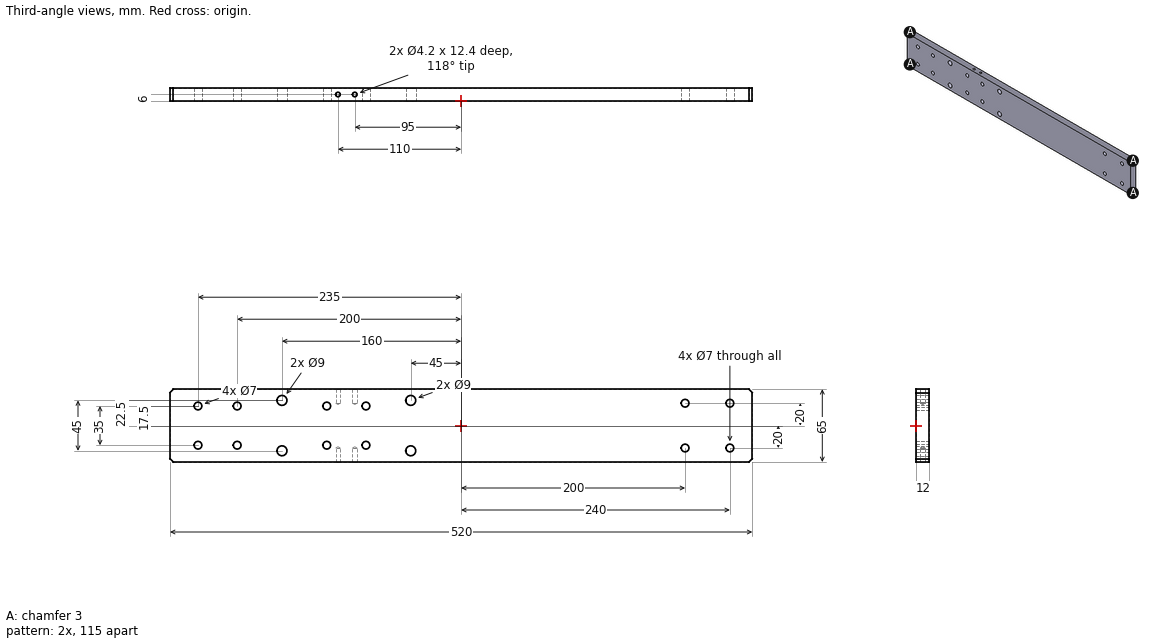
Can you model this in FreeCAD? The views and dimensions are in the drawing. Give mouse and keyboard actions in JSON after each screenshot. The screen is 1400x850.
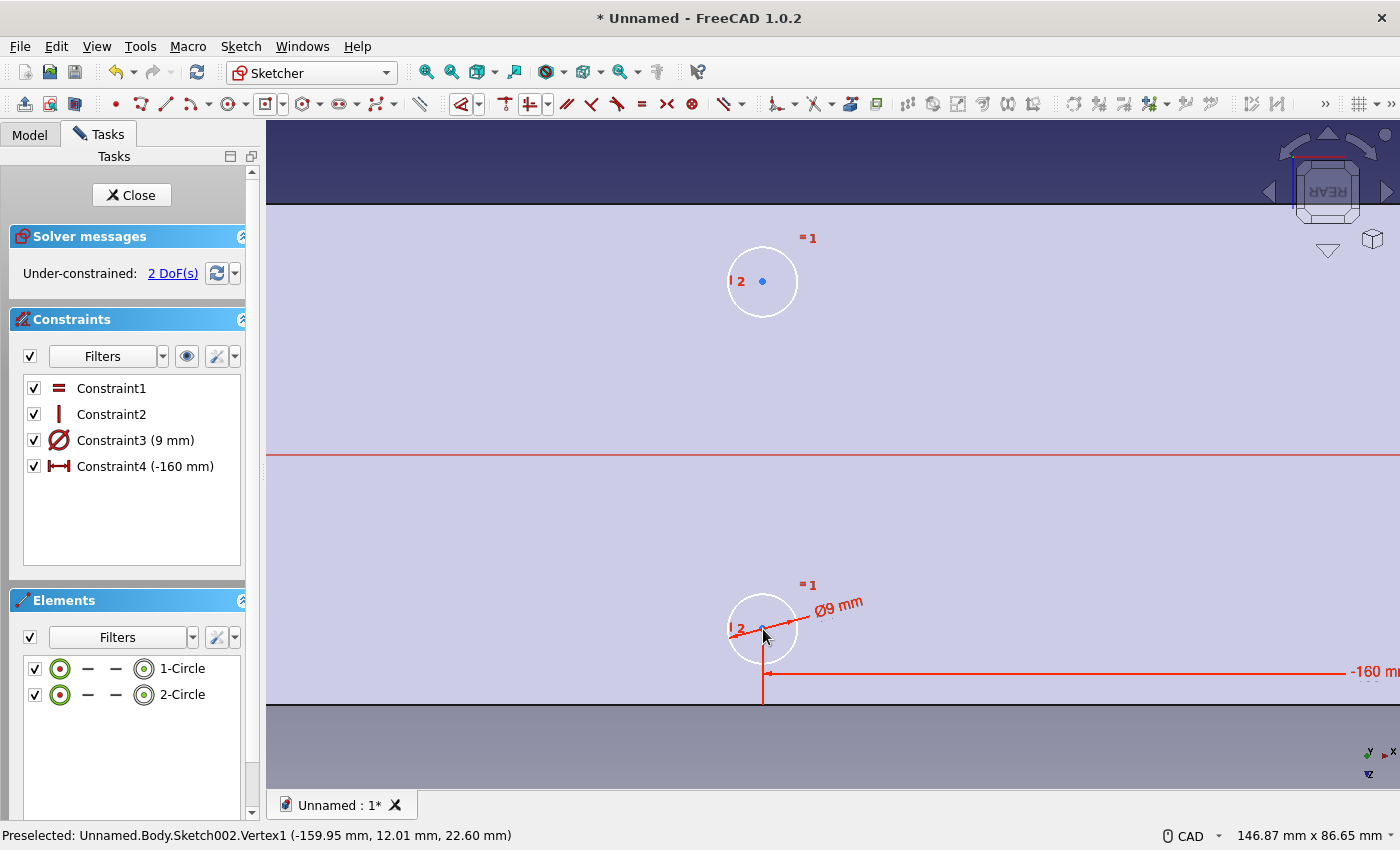
{"action": "left_click", "coordinate": [763, 629]}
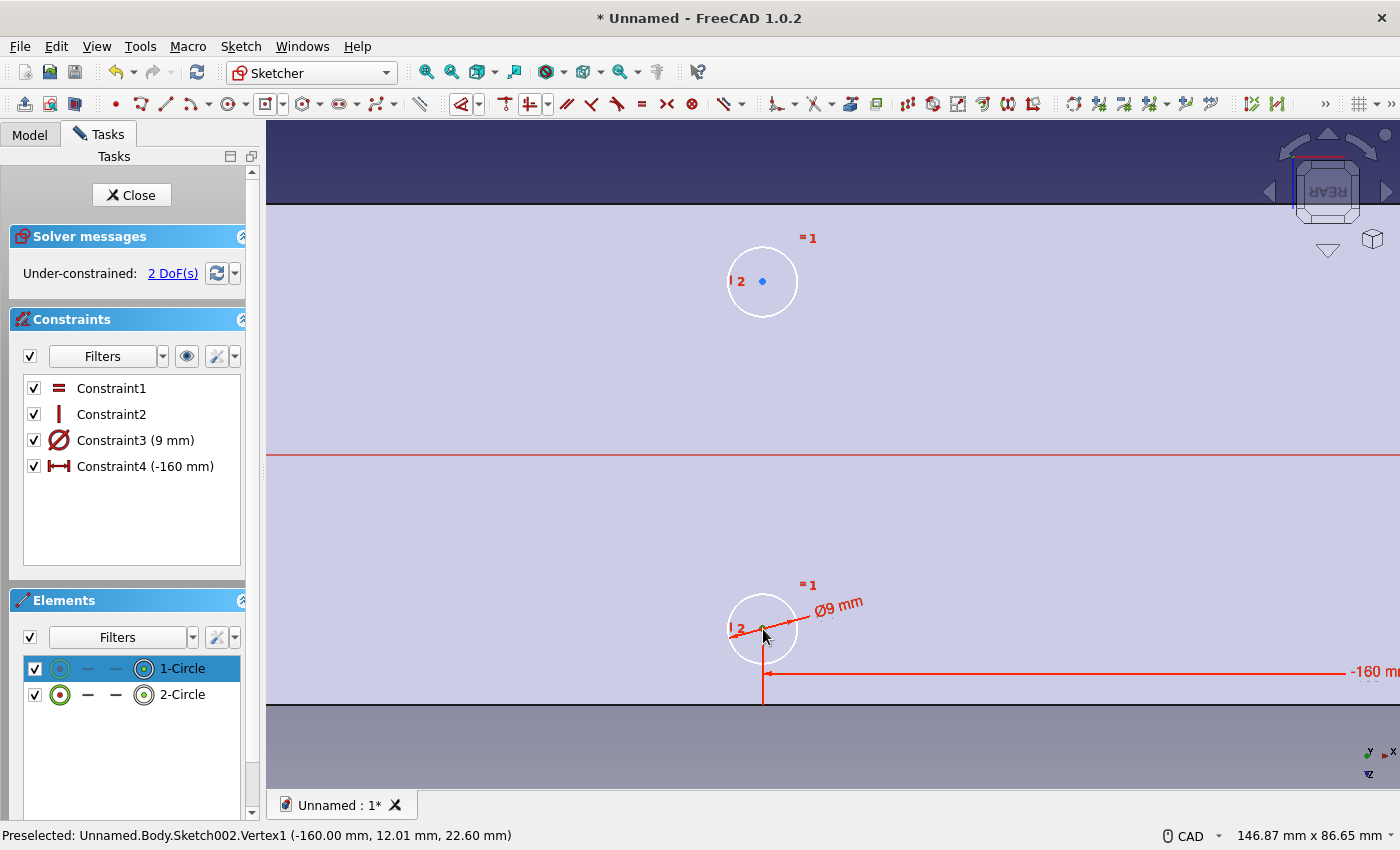
{"action": "left_click", "coordinate": [763, 282]}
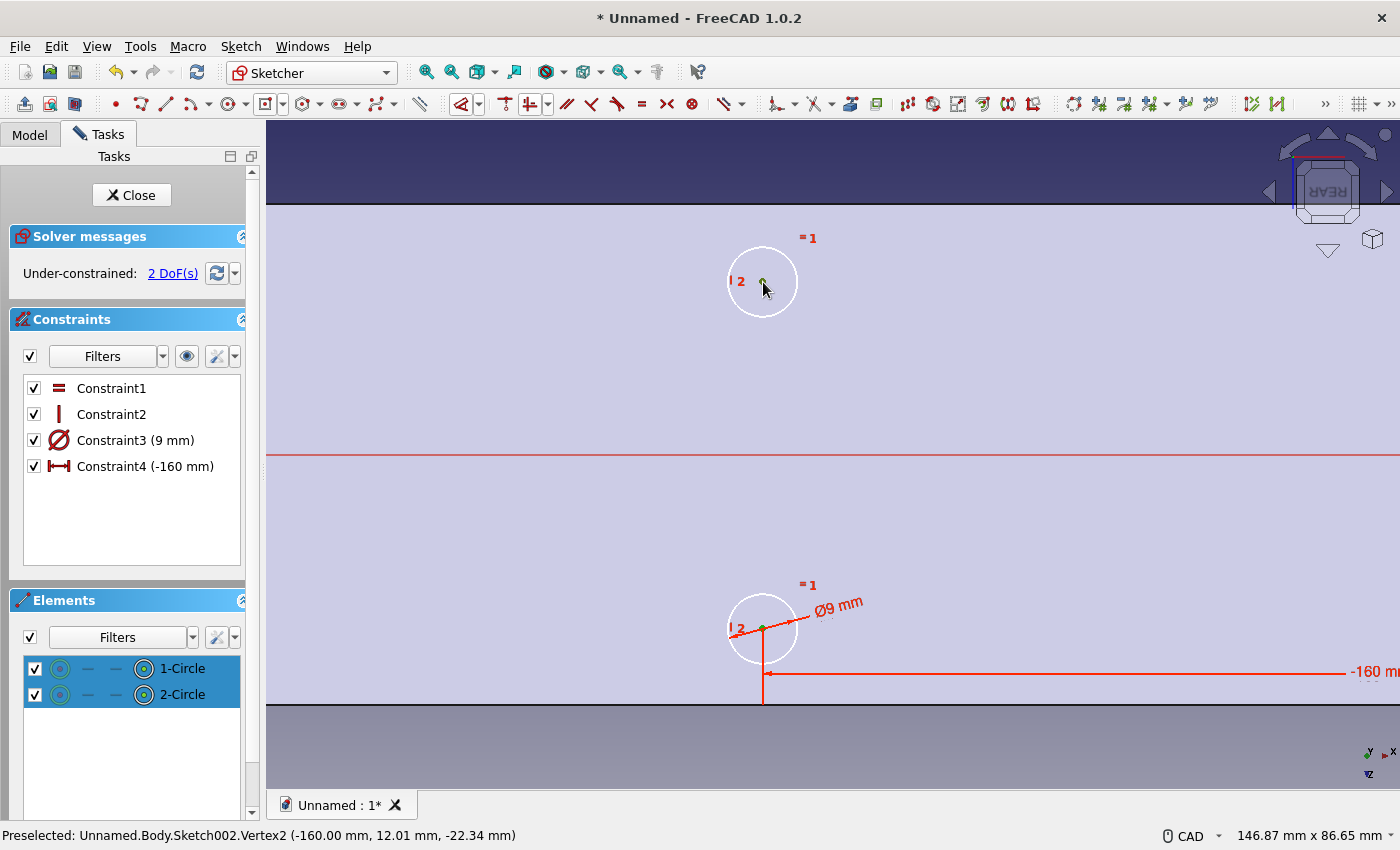
{"action": "left_click", "coordinate": [478, 104]}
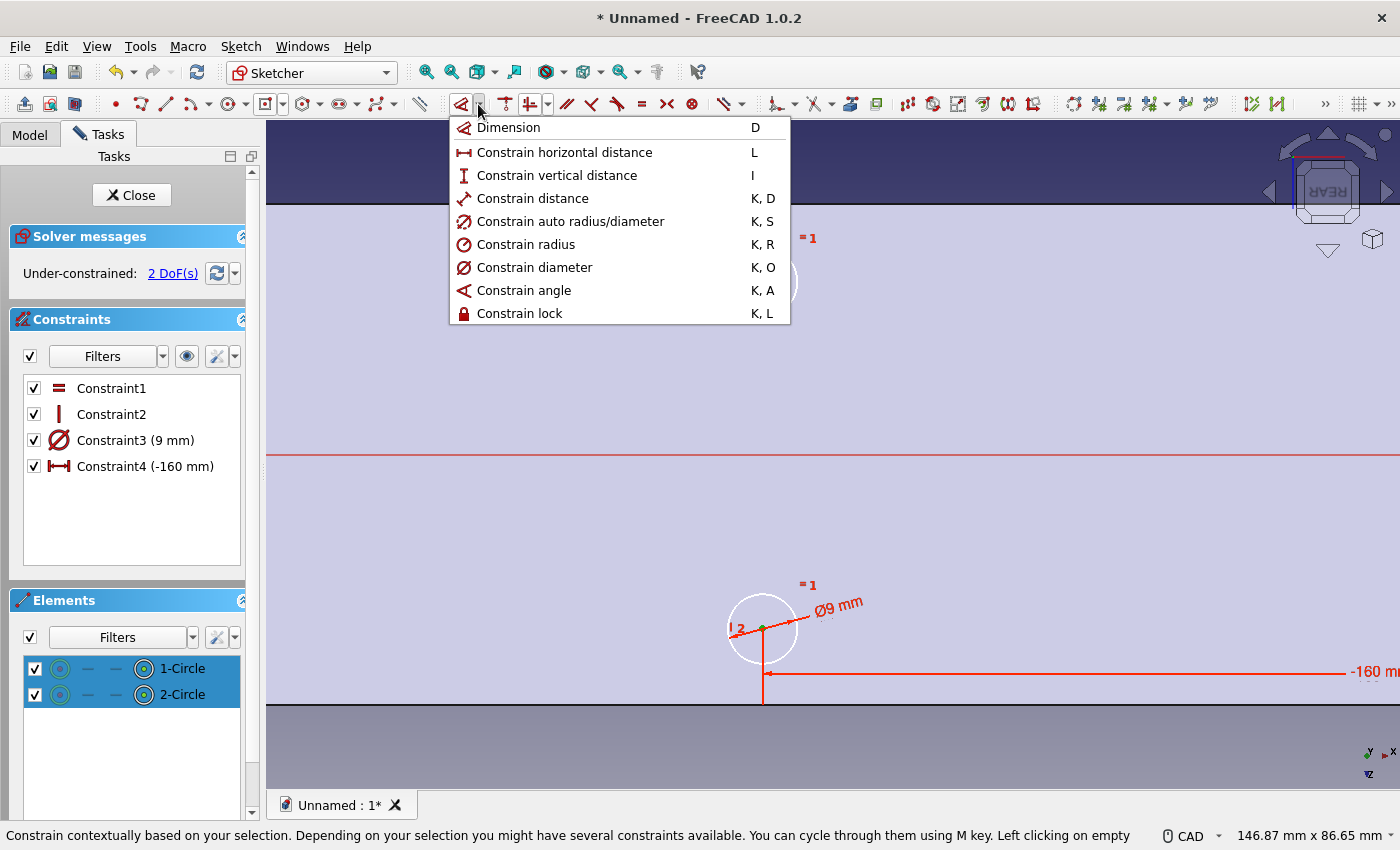
{"action": "left_click", "coordinate": [620, 176]}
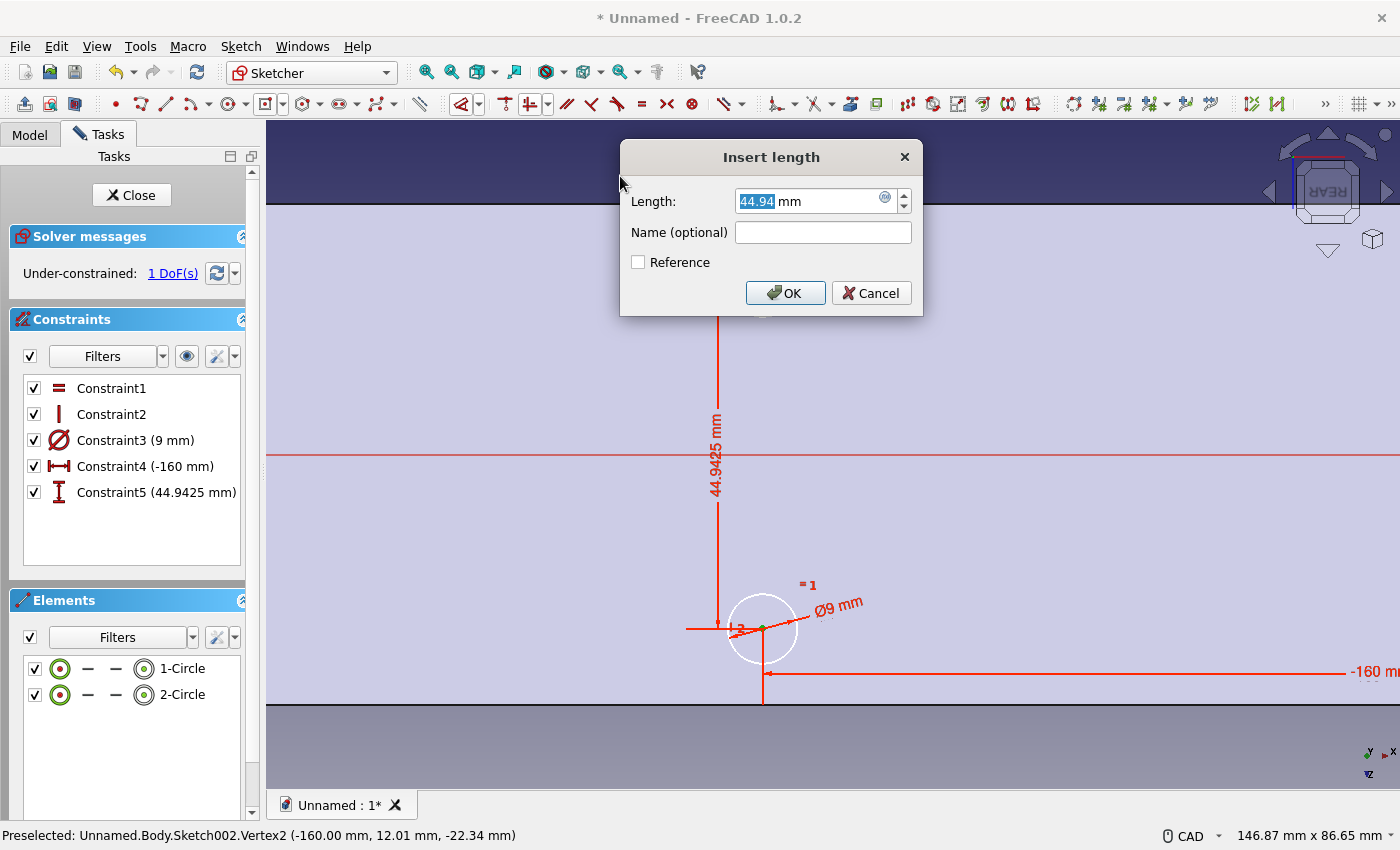
{"action": "type", "text": "45"}
{"action": "key", "text": "Return"}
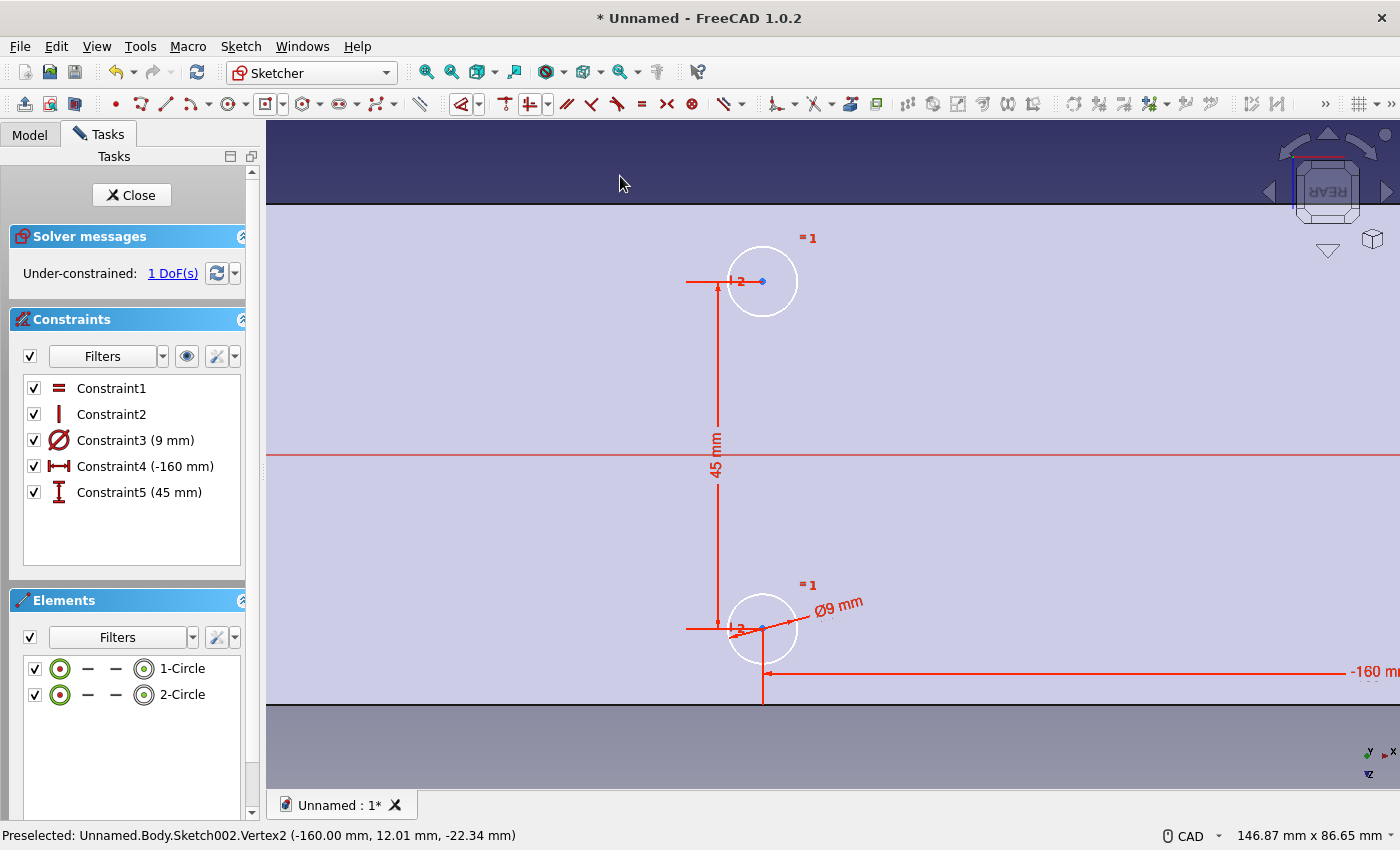
{"action": "left_click", "coordinate": [763, 629]}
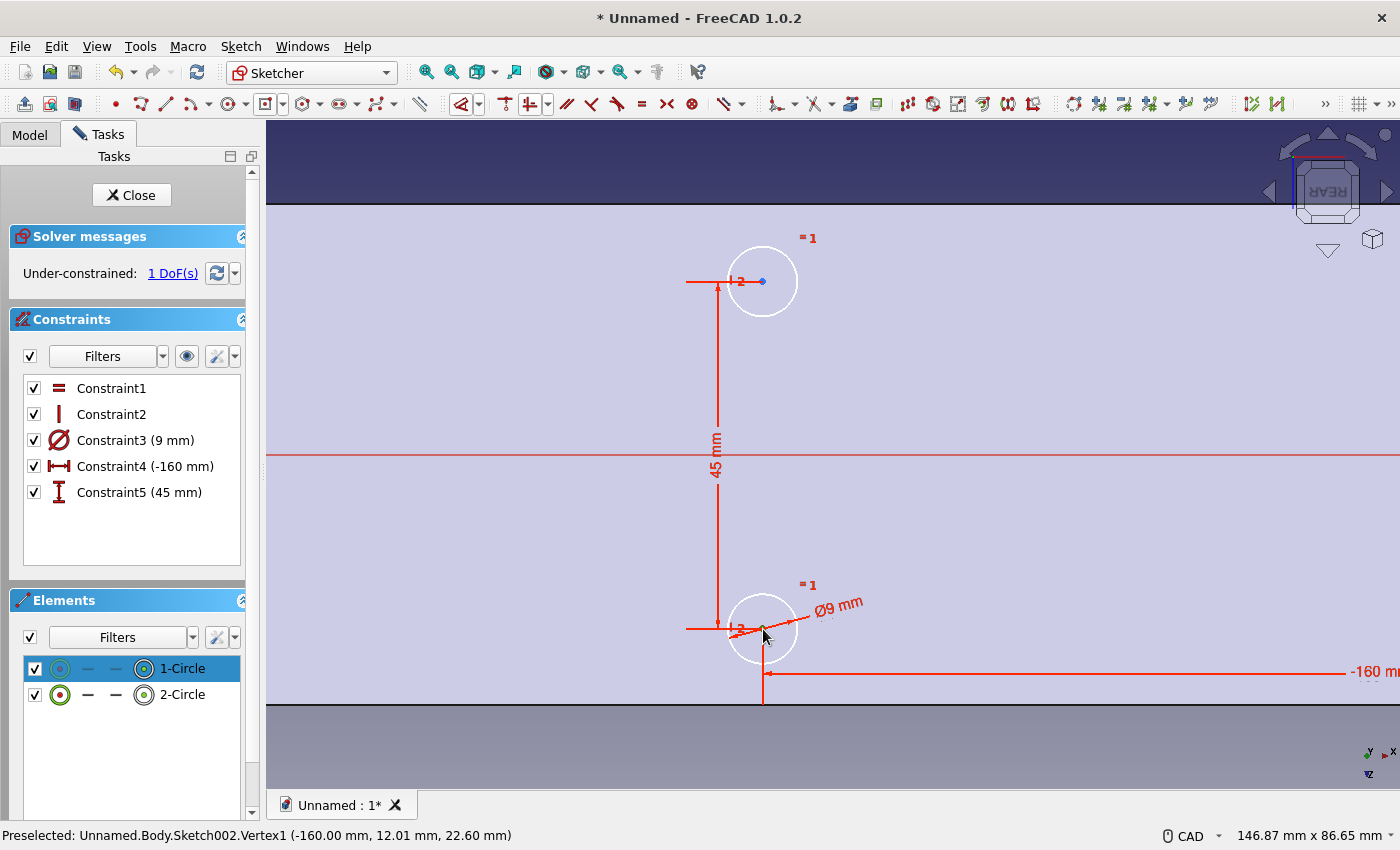
{"action": "key", "text": "i"}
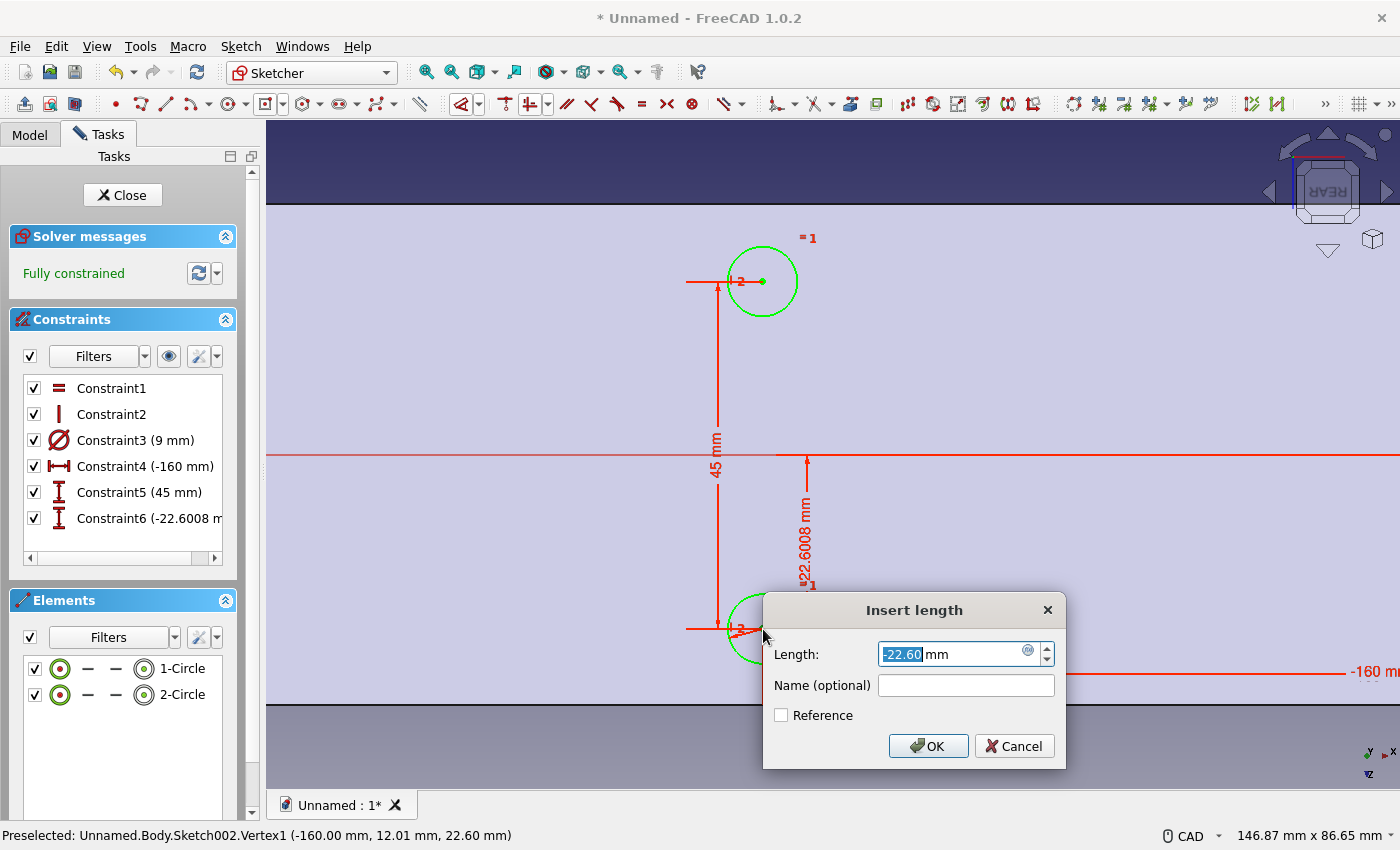
{"action": "type", "text": "-22.5"}
{"action": "key", "text": "Return"}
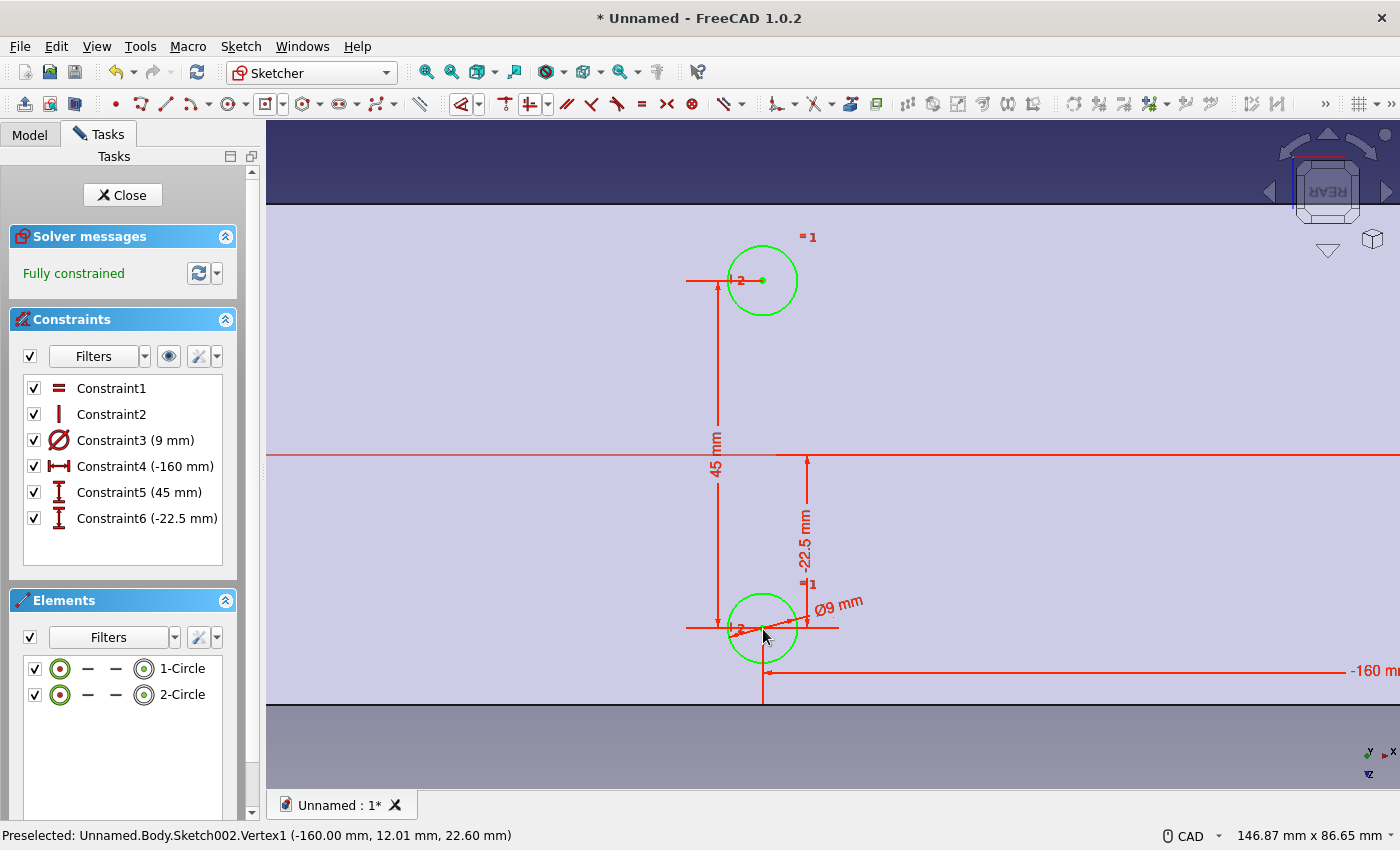
{"action": "left_click", "coordinate": [123, 195]}